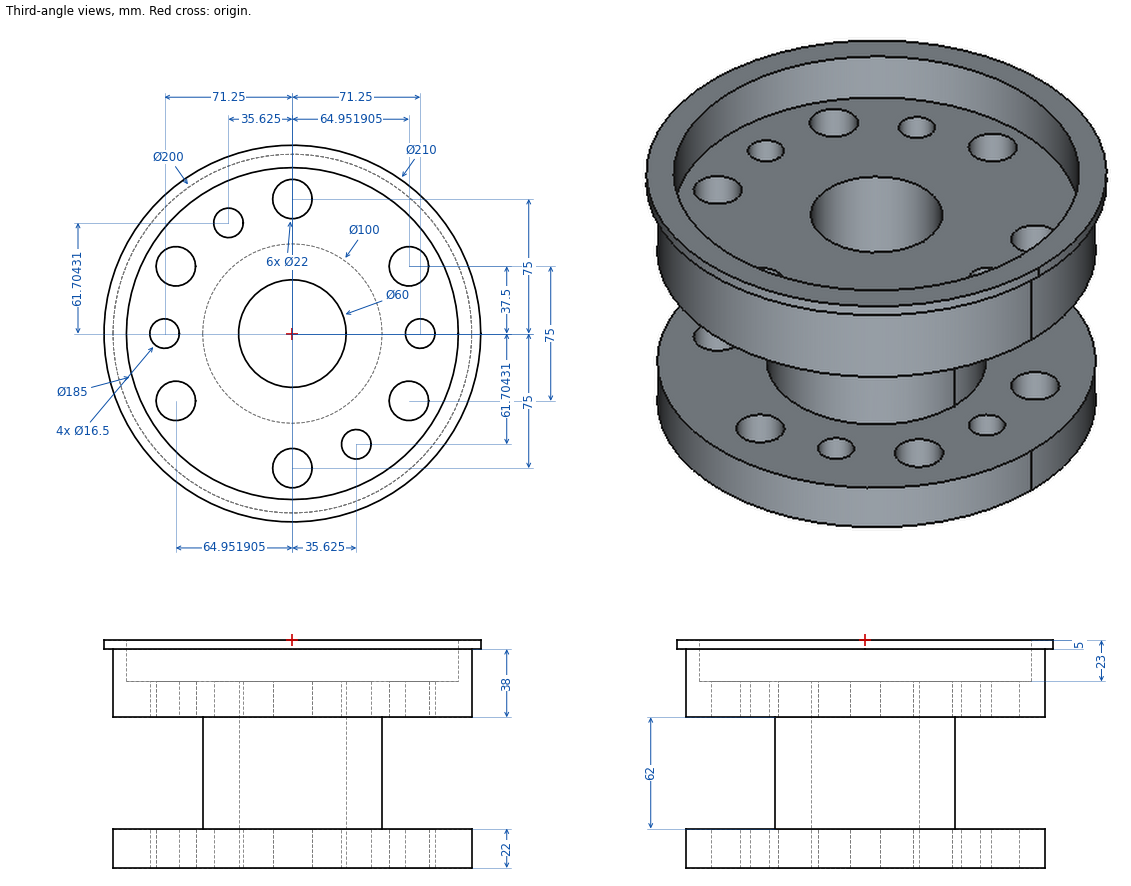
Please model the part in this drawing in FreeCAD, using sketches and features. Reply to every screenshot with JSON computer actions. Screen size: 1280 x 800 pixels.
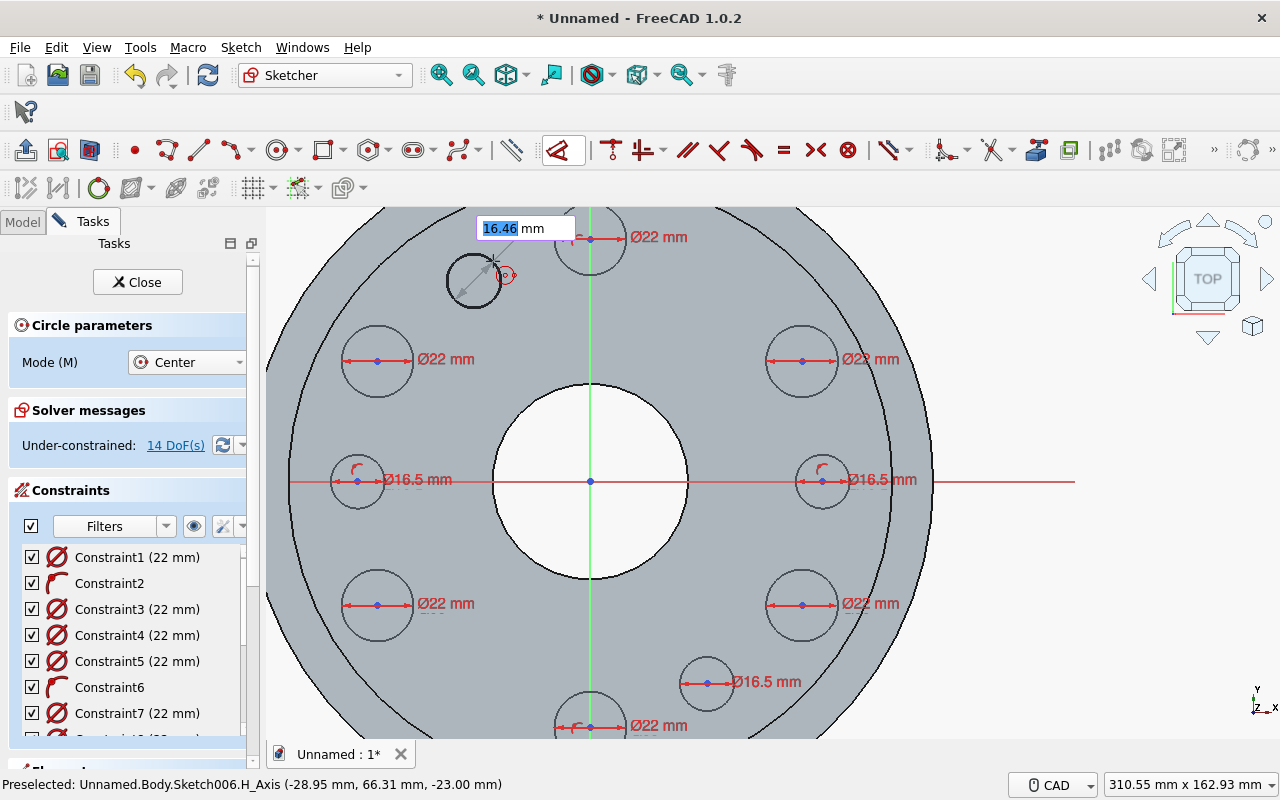
{"action": "type", "text": "16.5"}
{"action": "key", "text": "Return"}
{"action": "key", "text": "Escape"}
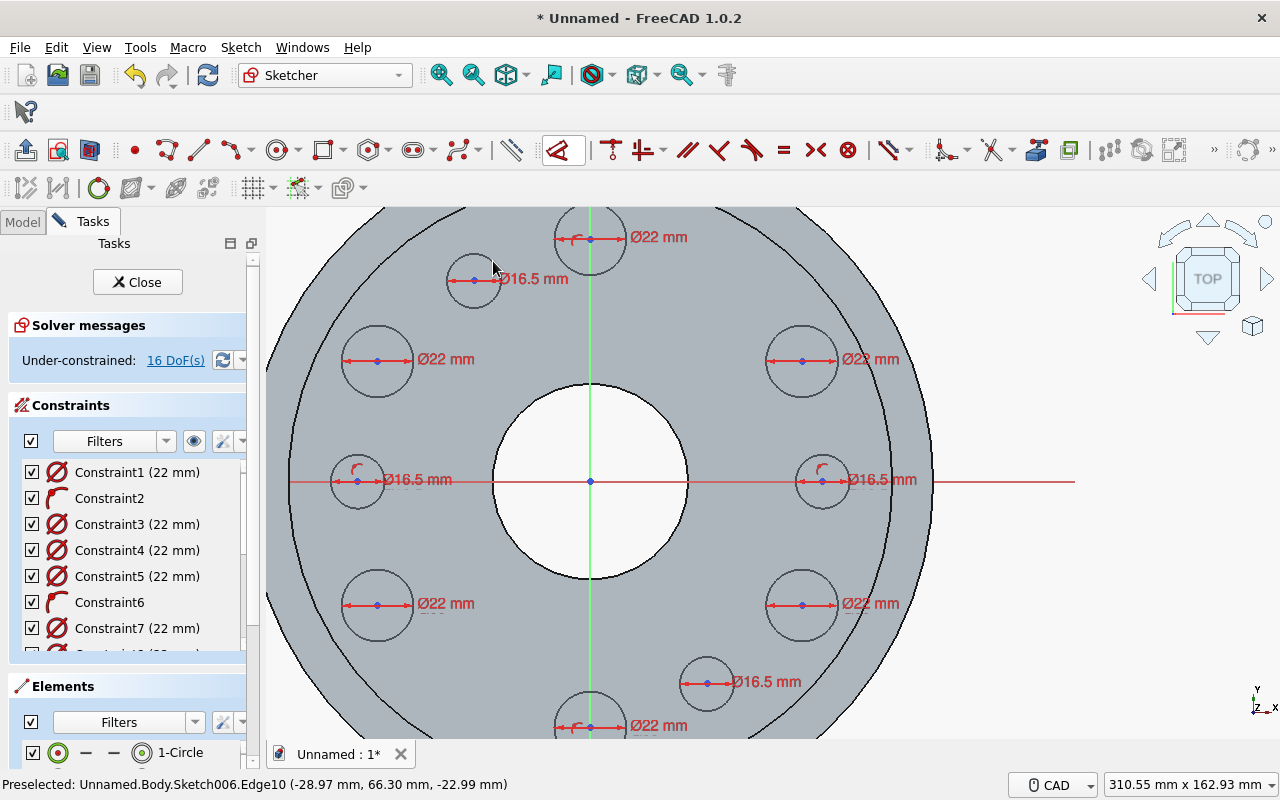
{"action": "left_click", "coordinate": [802, 361]}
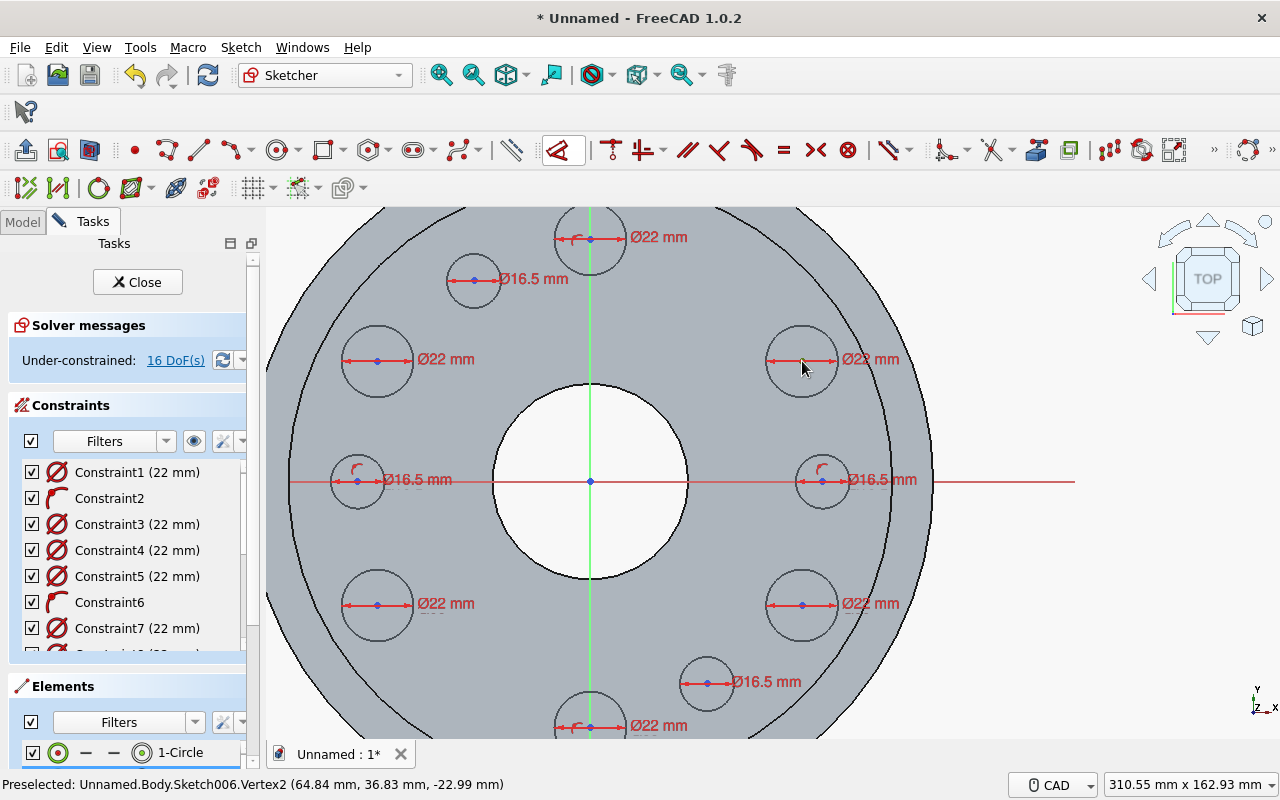
{"action": "left_click", "coordinate": [802, 606]}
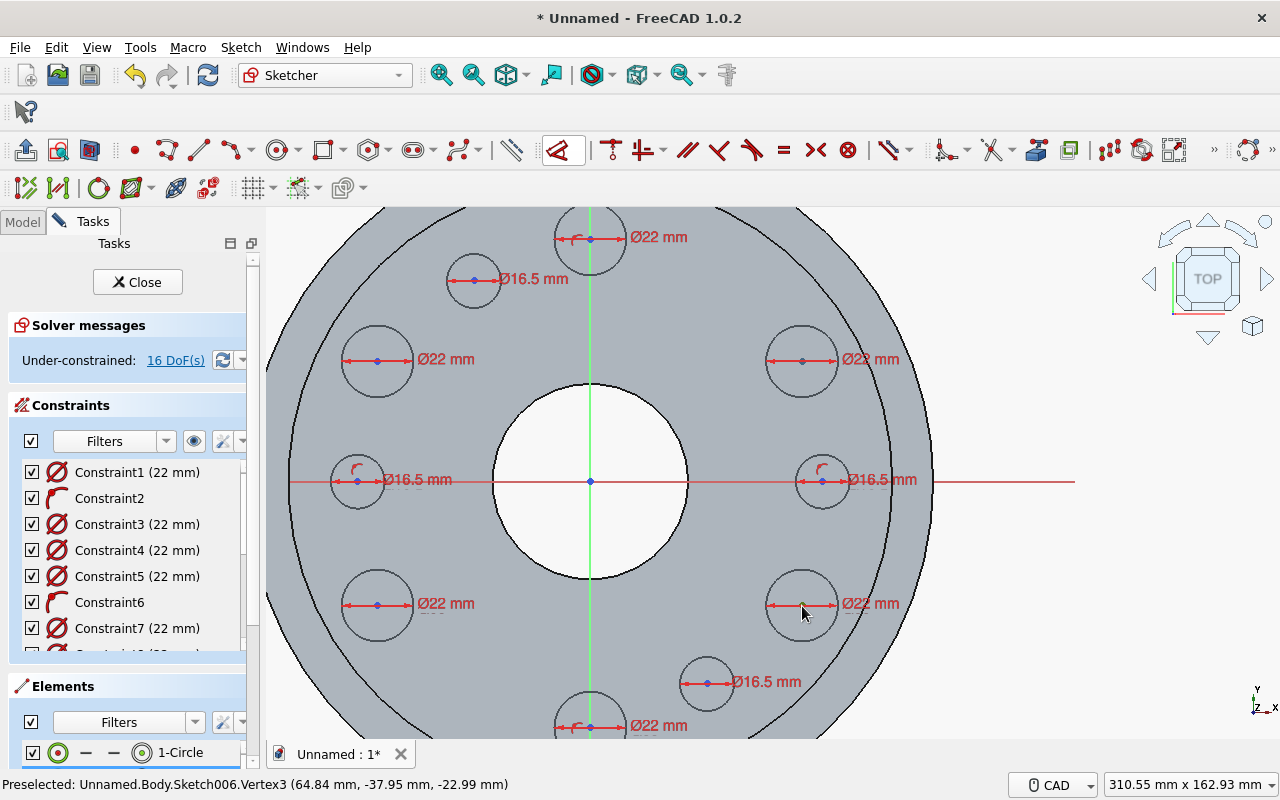
{"action": "key", "text": "v"}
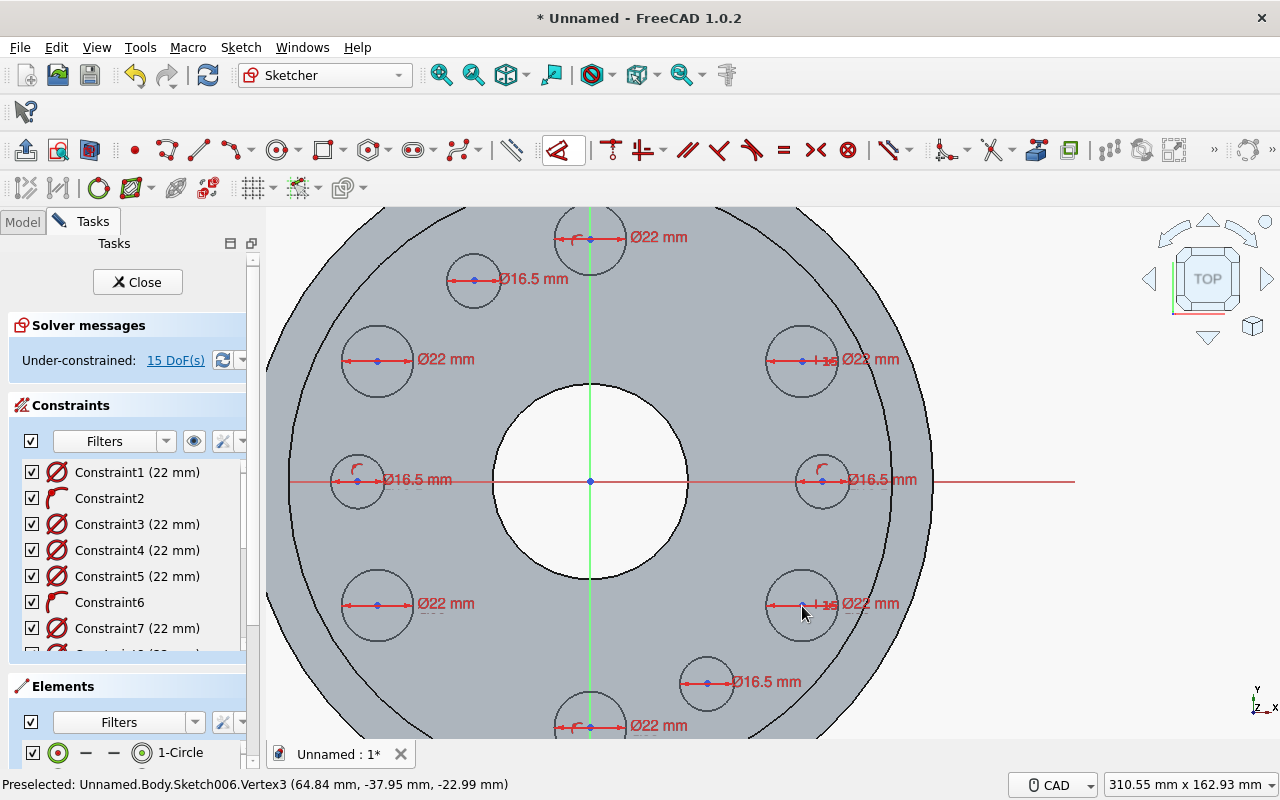
{"action": "left_click", "coordinate": [802, 606]}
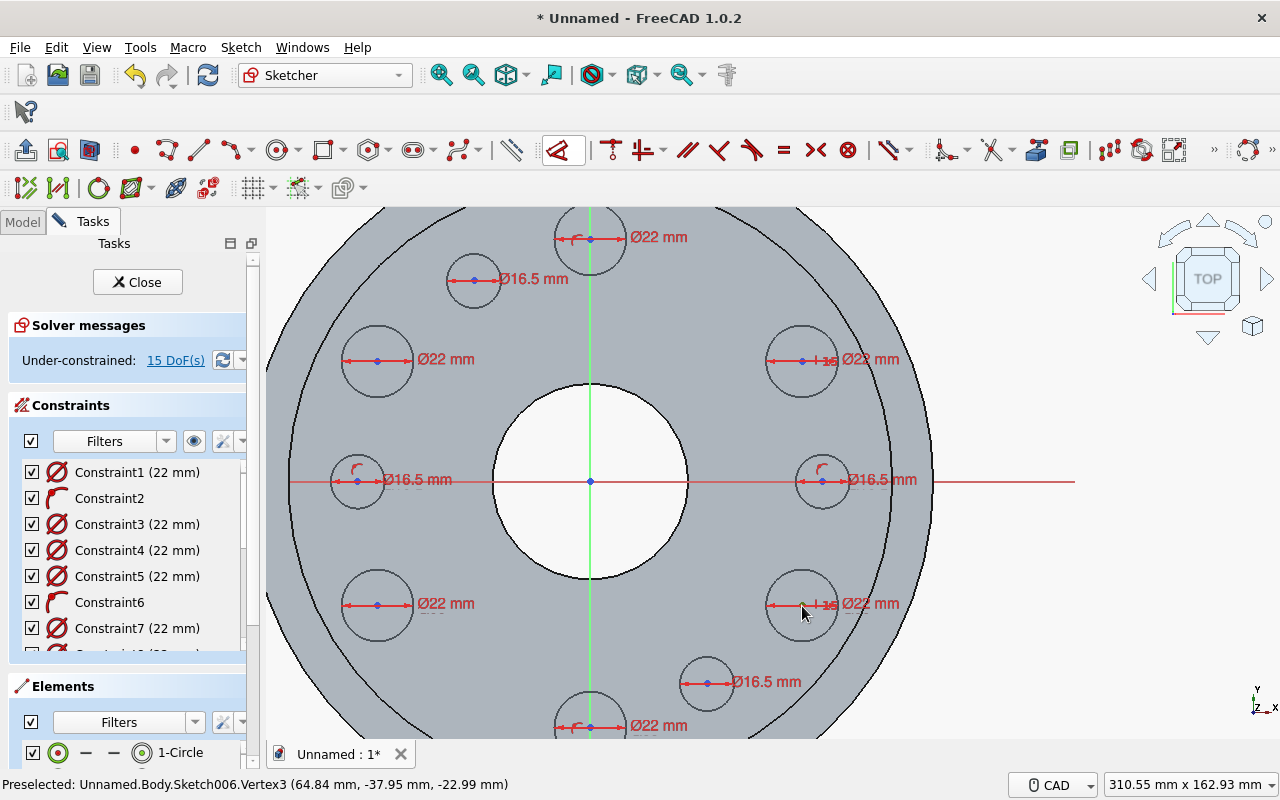
{"action": "left_click", "coordinate": [378, 606]}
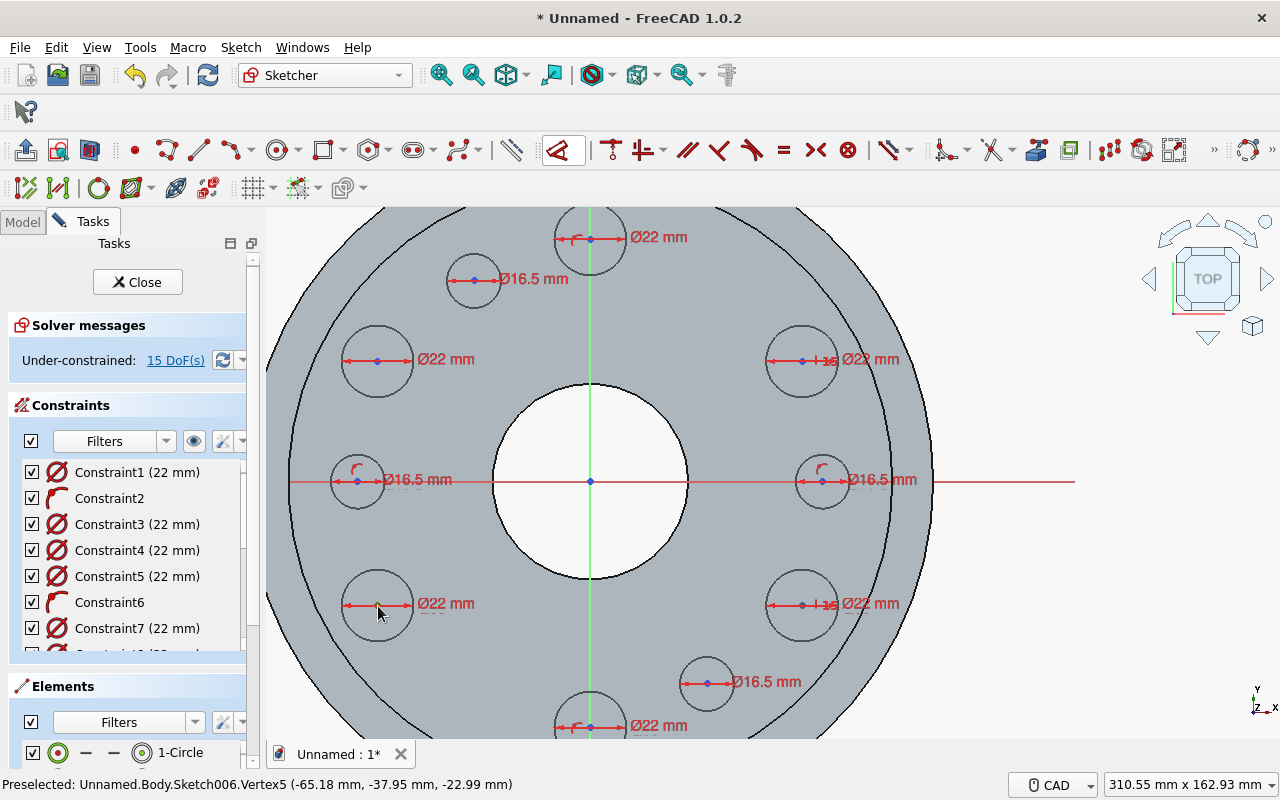
{"action": "key", "text": "h"}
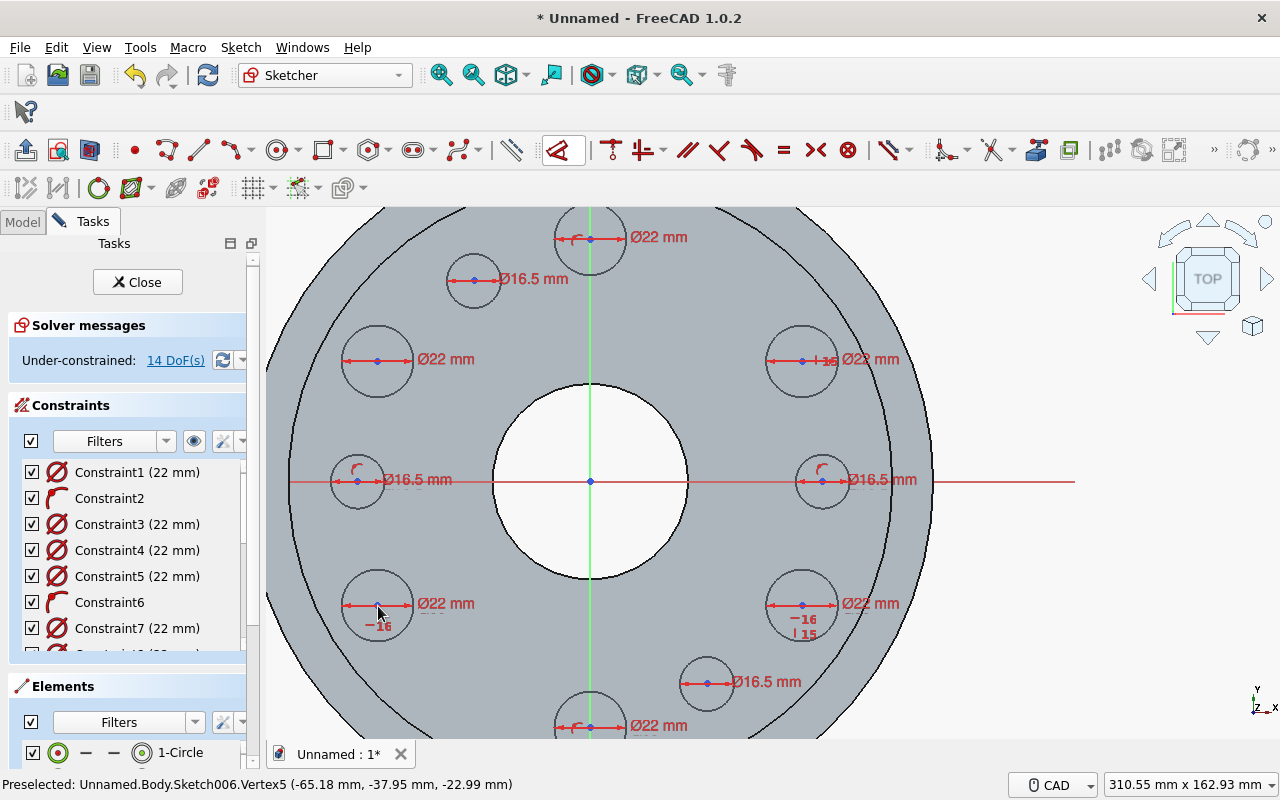
{"action": "left_click", "coordinate": [378, 606]}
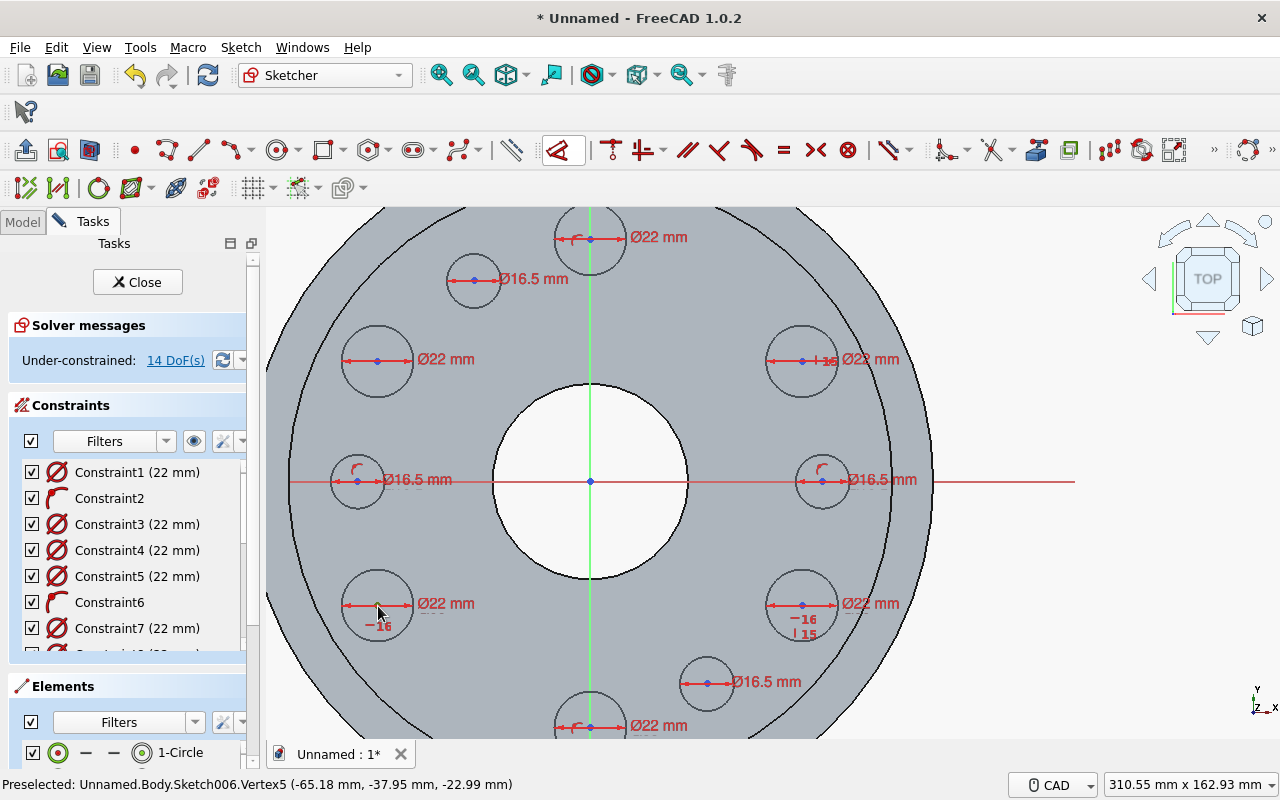
{"action": "left_click", "coordinate": [378, 361]}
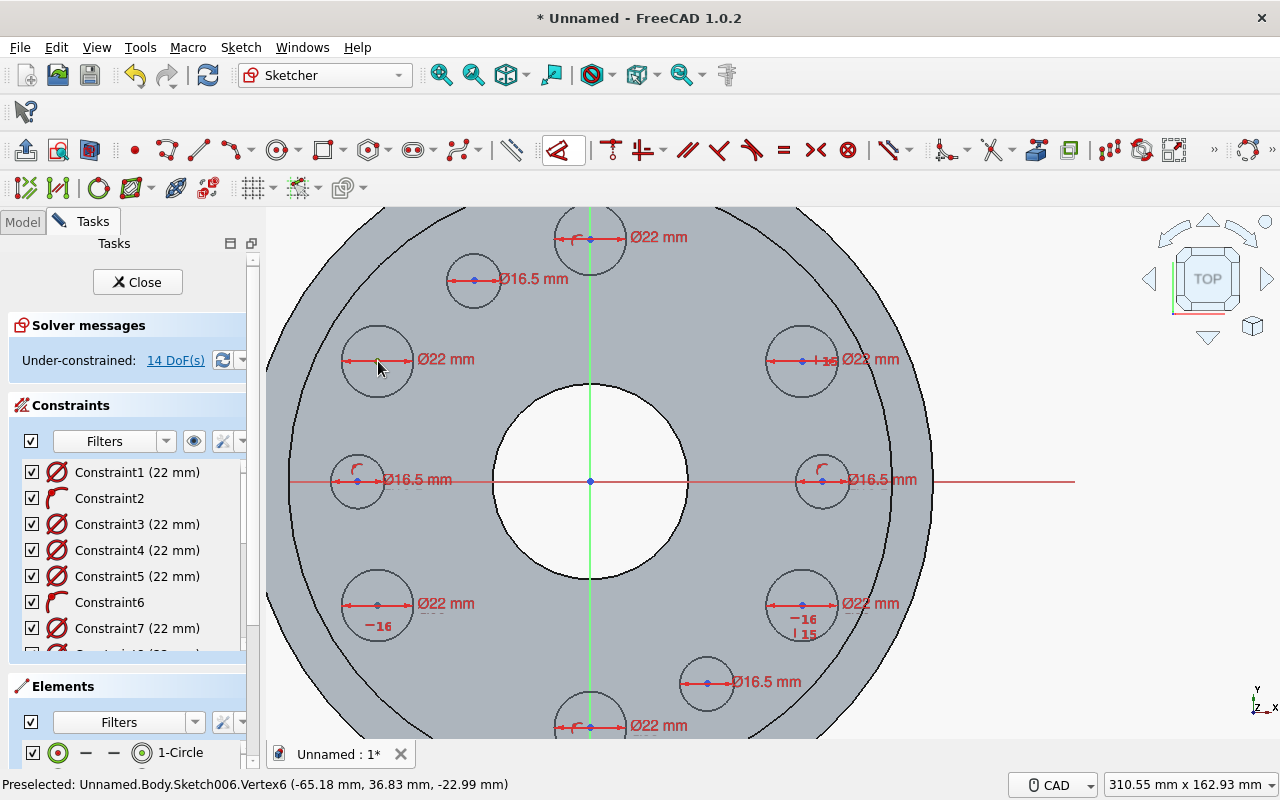
{"action": "left_click", "coordinate": [666, 150]}